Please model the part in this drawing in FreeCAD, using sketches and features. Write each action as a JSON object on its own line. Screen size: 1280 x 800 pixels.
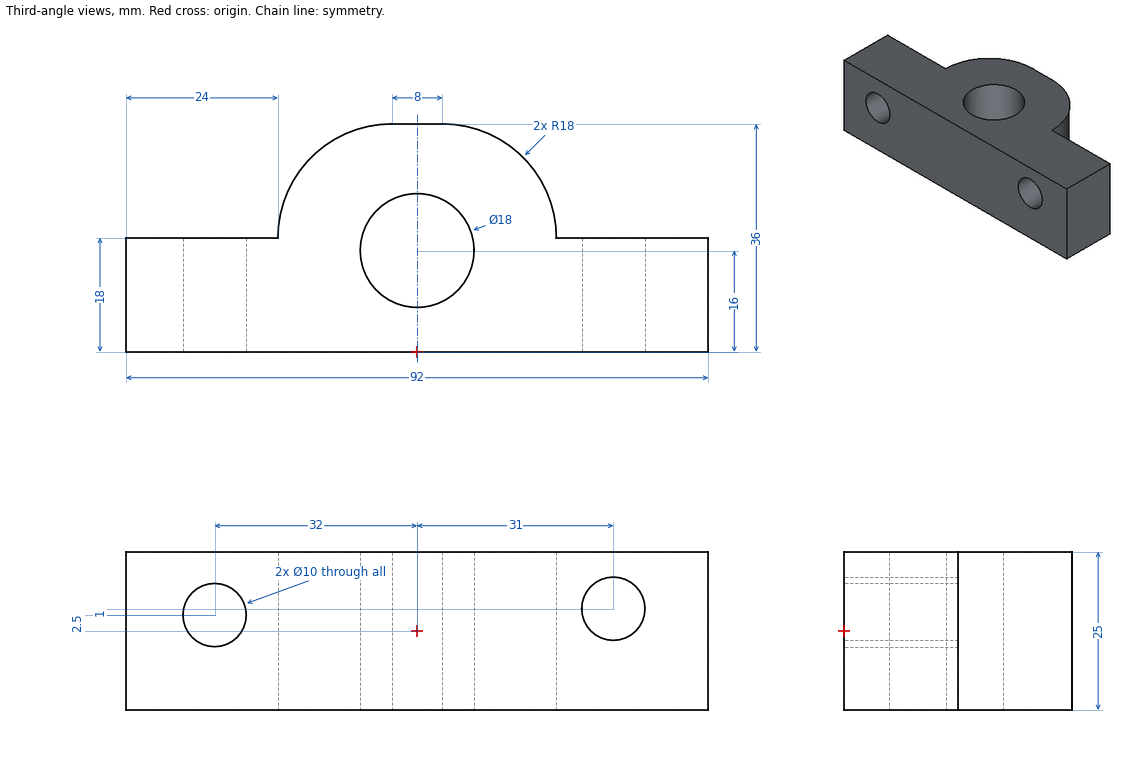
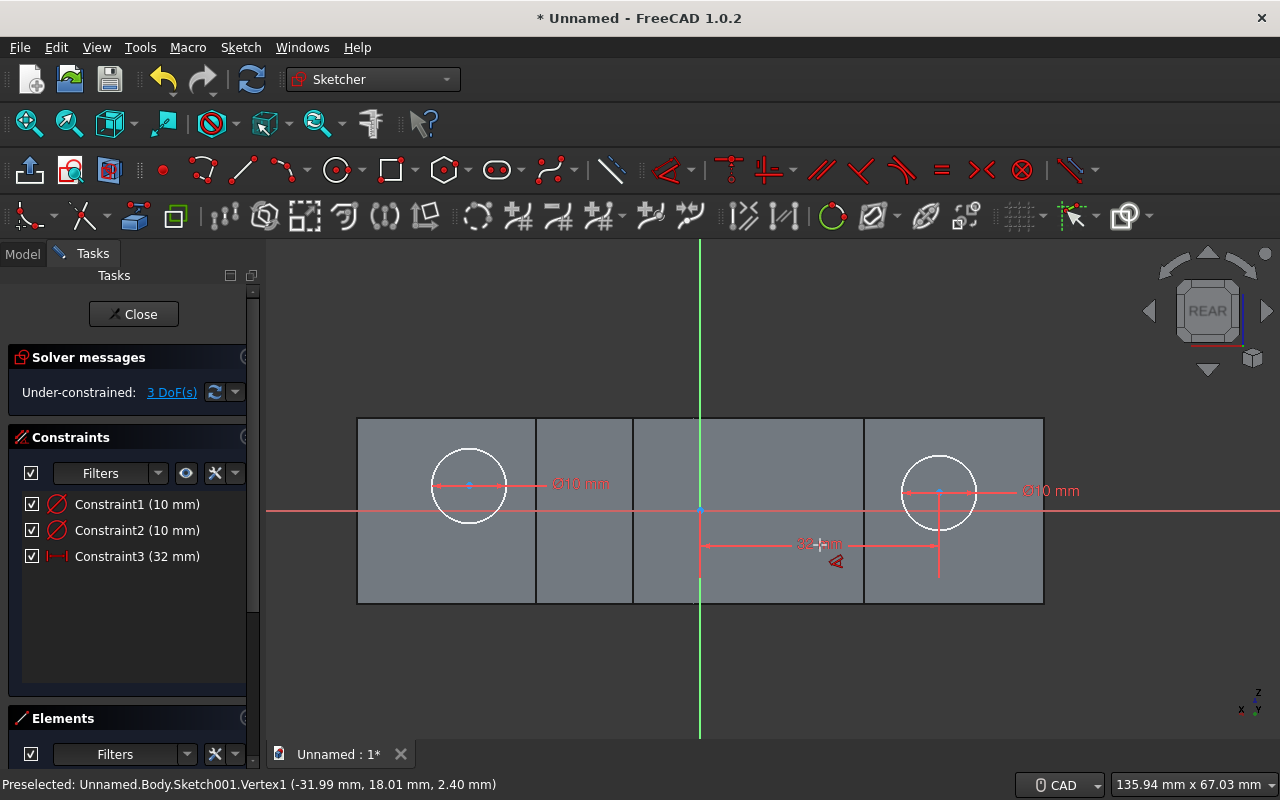
{"action": "left_click", "coordinate": [469, 486]}
{"action": "left_click", "coordinate": [585, 545]}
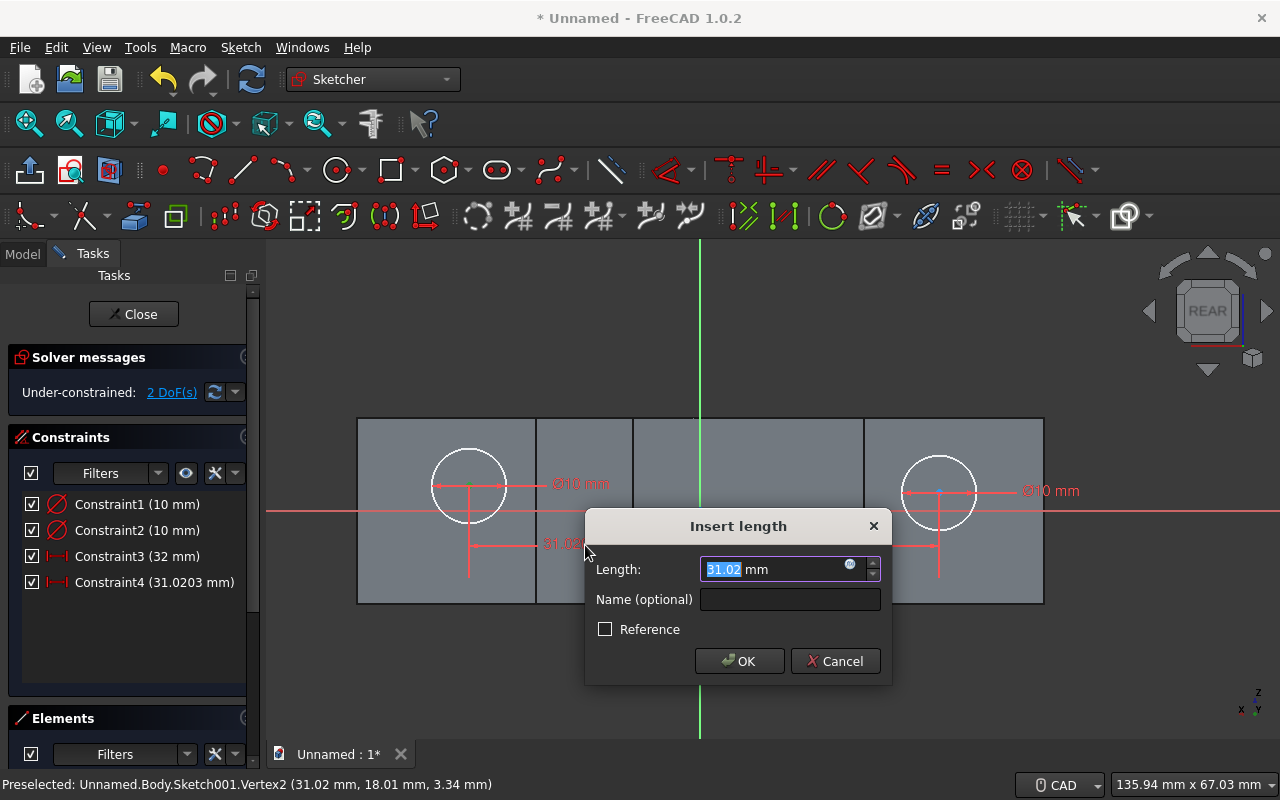
{"action": "type", "text": "31"}
{"action": "key", "text": "Return"}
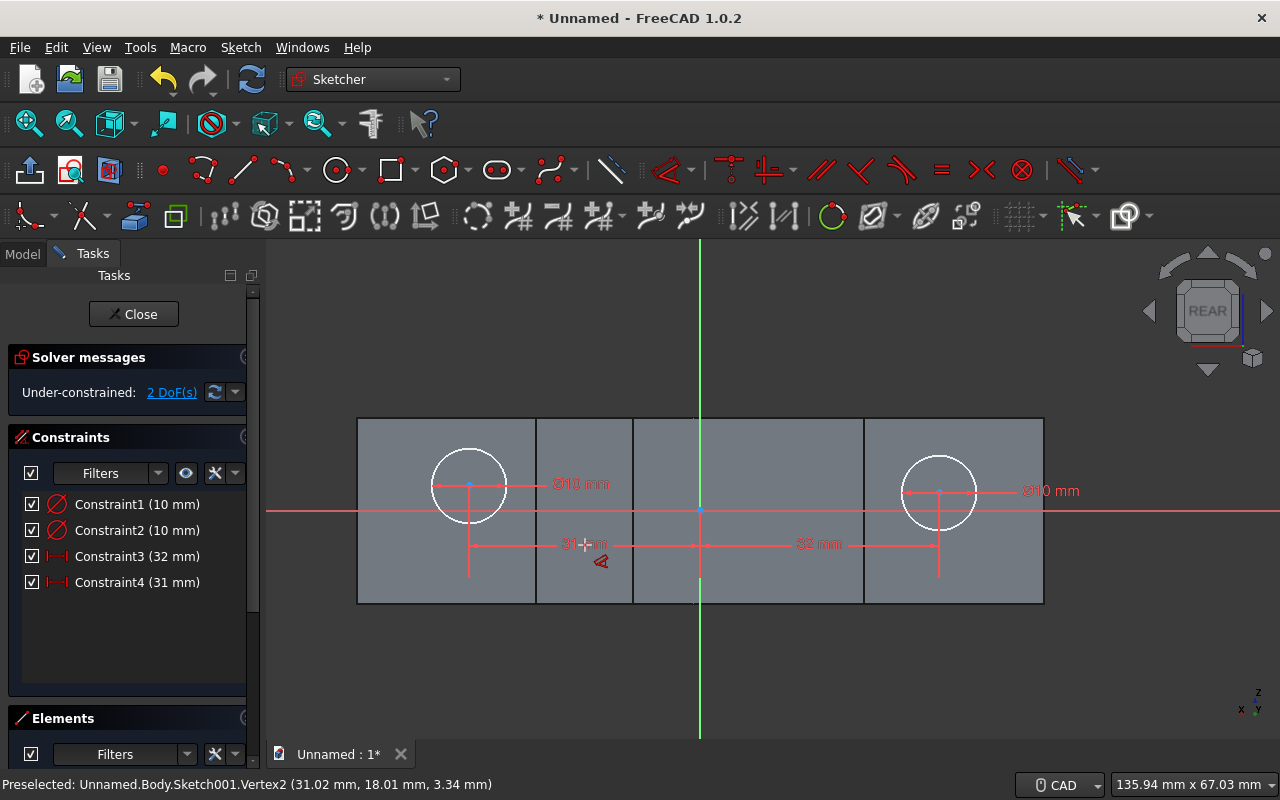
{"action": "scroll", "coordinate": [939, 493], "scroll_direction": "up", "scroll_amount": 9}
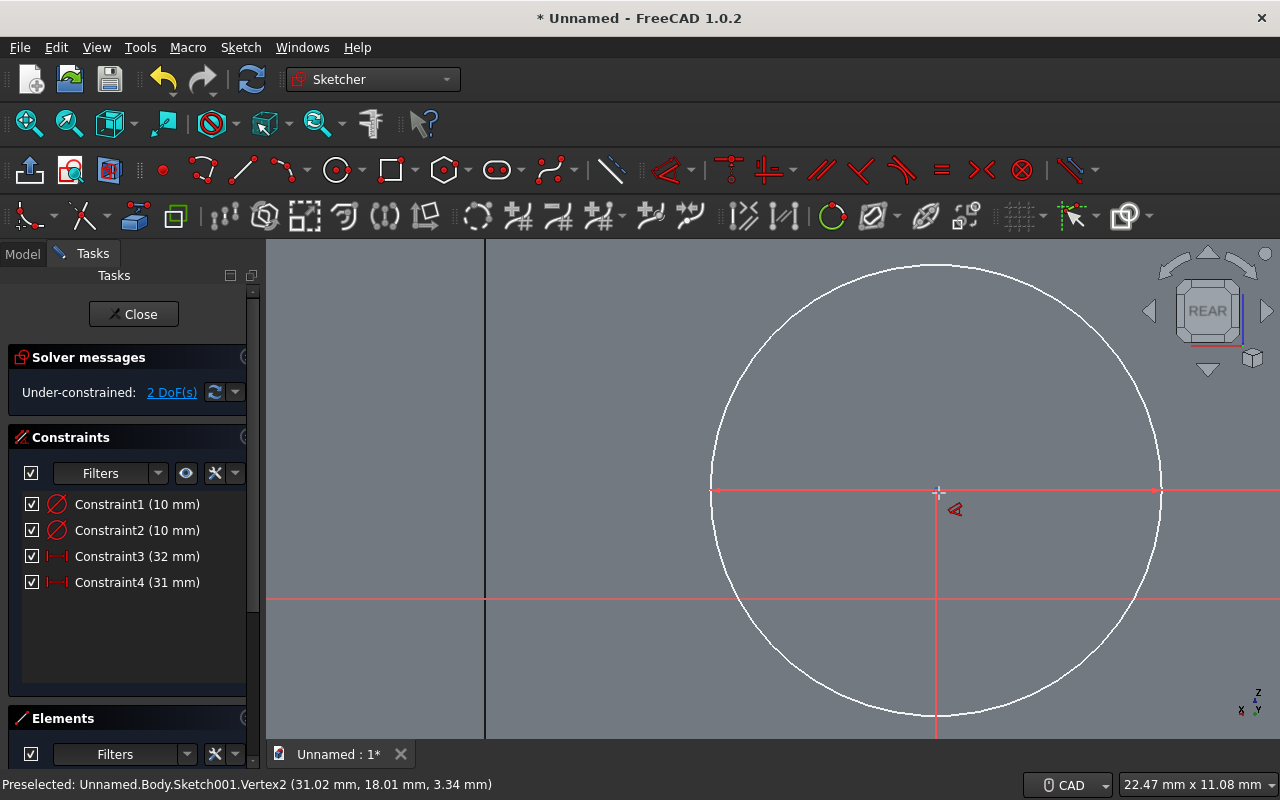
{"action": "left_click", "coordinate": [936, 490]}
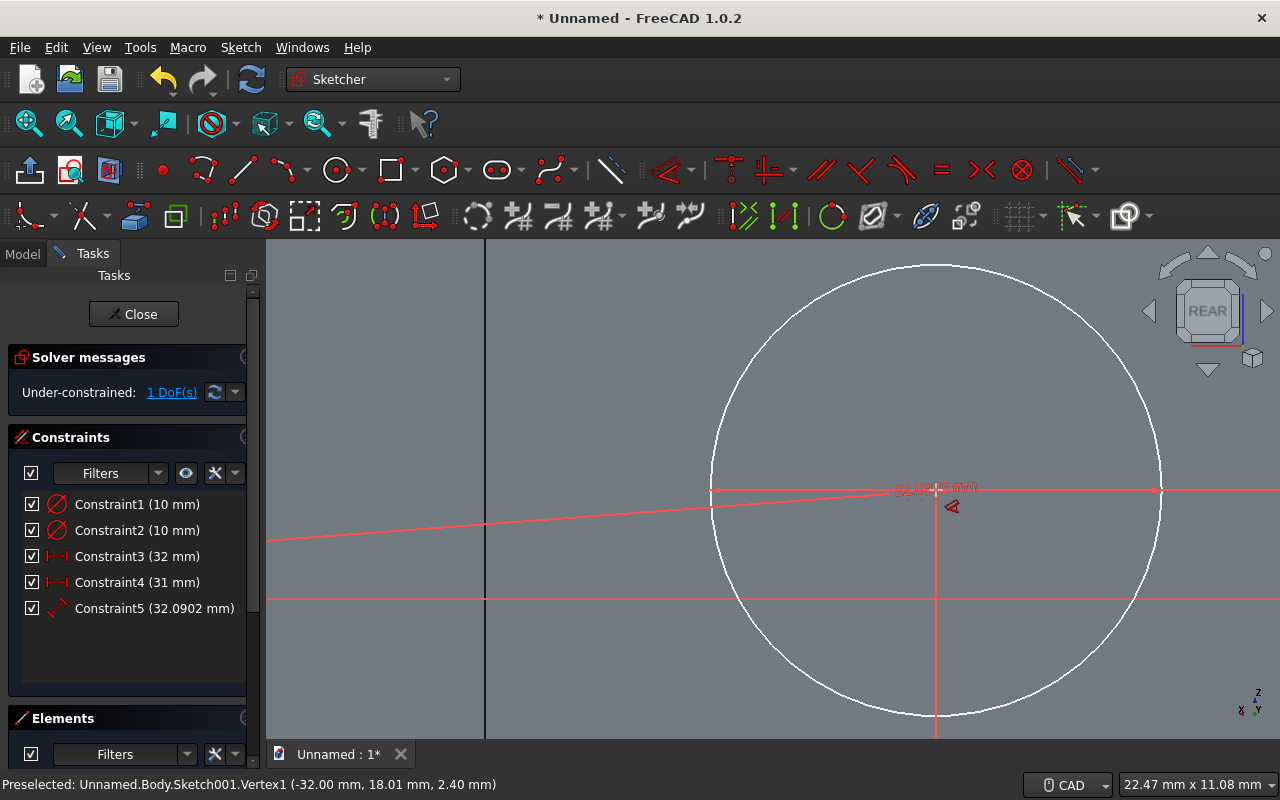
{"action": "scroll", "coordinate": [940, 494], "scroll_direction": "down", "scroll_amount": 9}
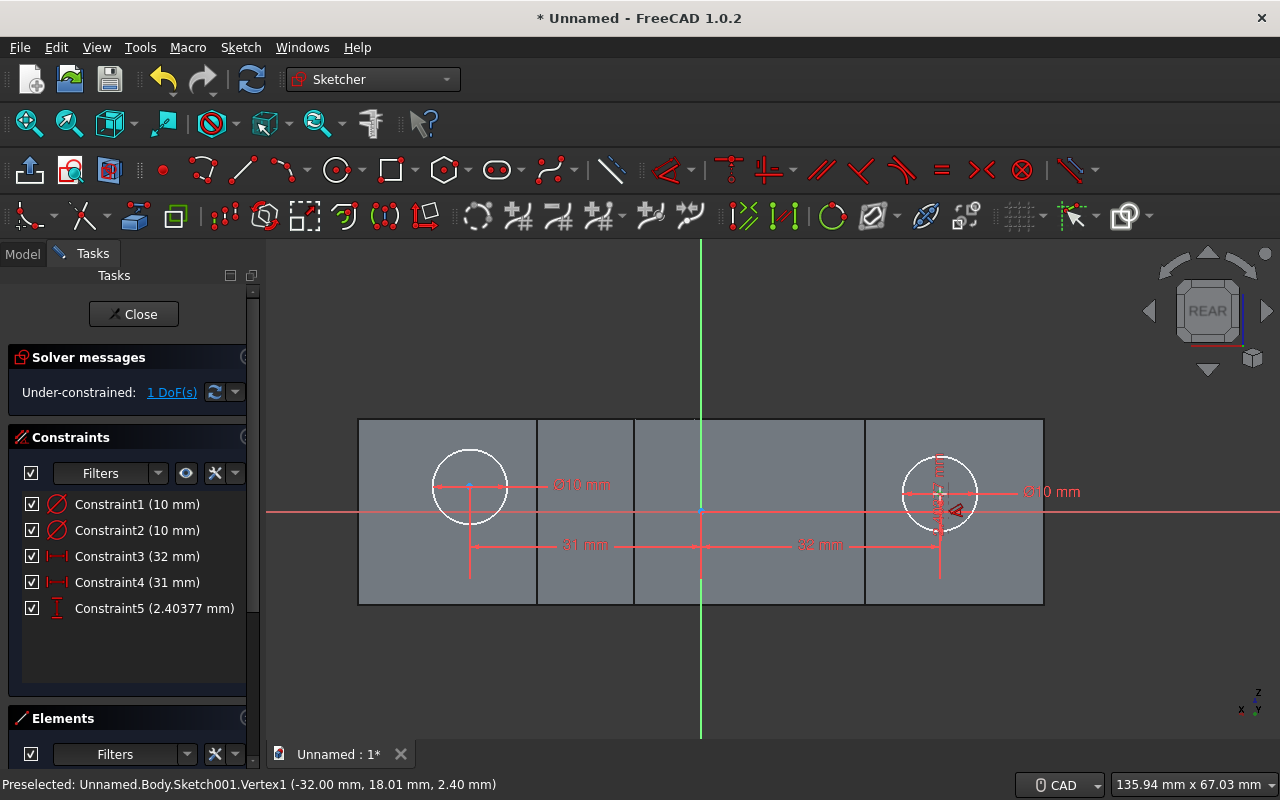
{"action": "scroll", "coordinate": [470, 487], "scroll_direction": "up", "scroll_amount": 9}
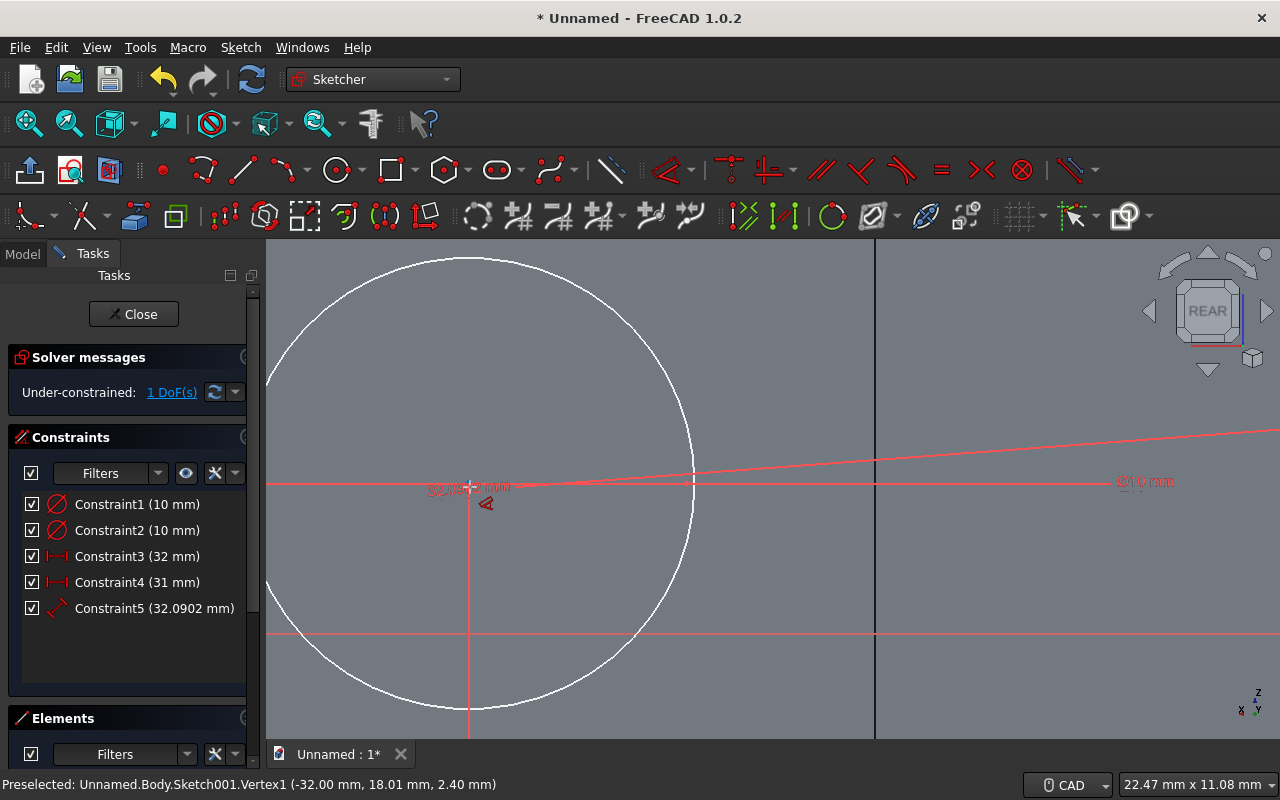
{"action": "left_click", "coordinate": [469, 484]}
{"action": "left_click", "coordinate": [435, 505]}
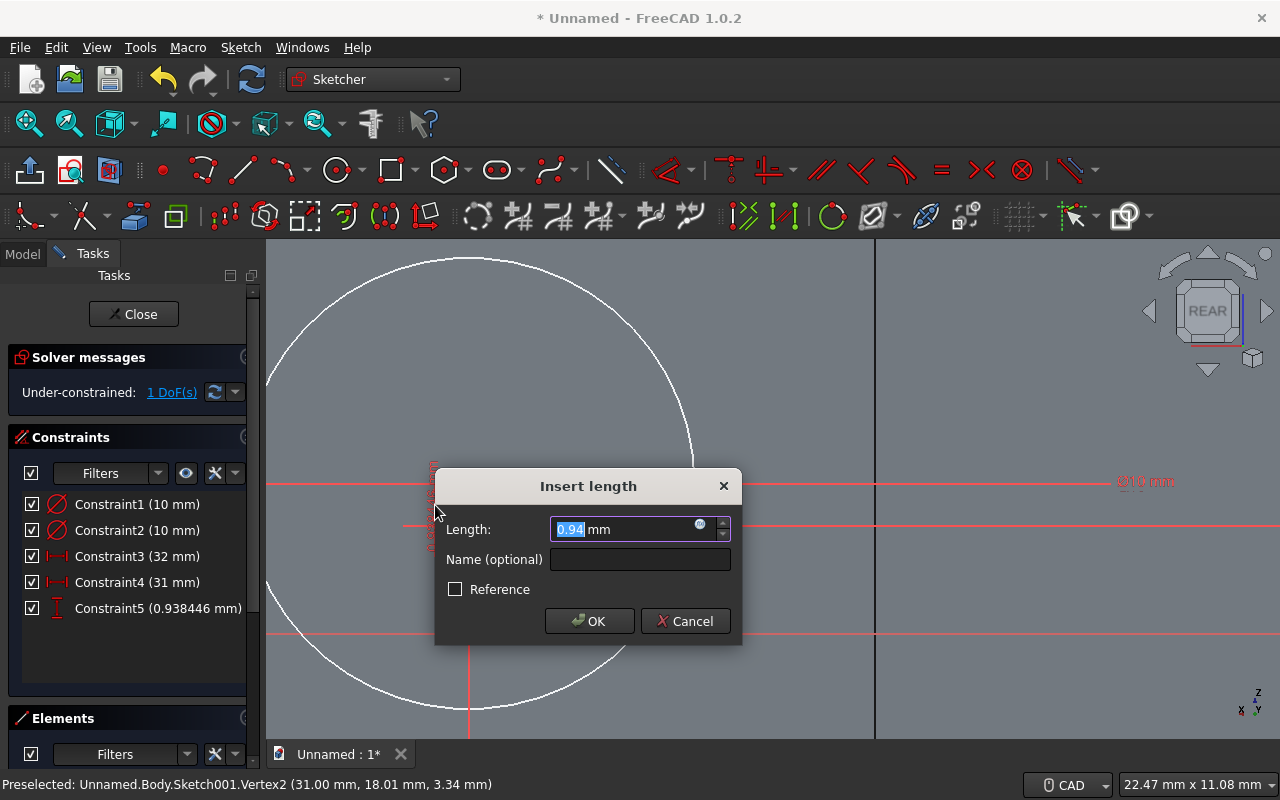
{"action": "type", "text": "1"}
{"action": "key", "text": "Return"}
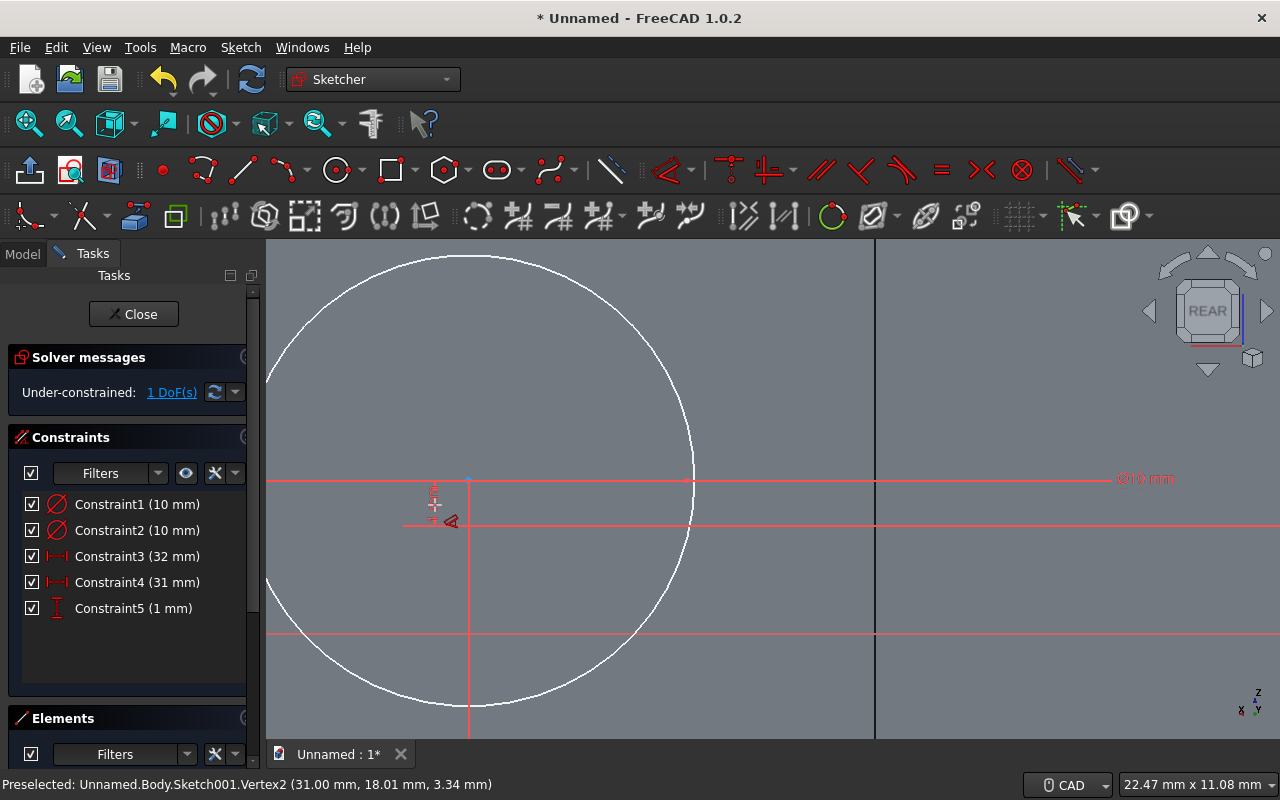
{"action": "scroll", "coordinate": [470, 487], "scroll_direction": "down", "scroll_amount": 9}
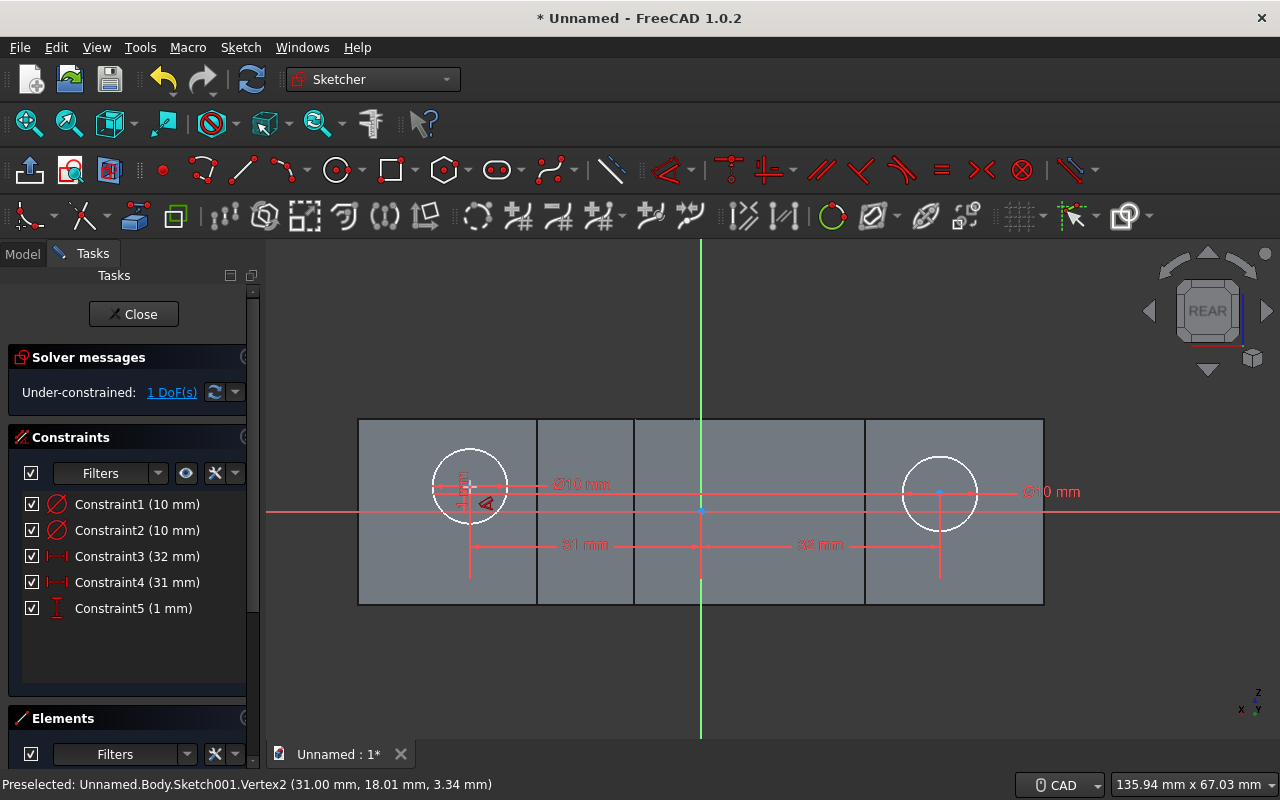
{"action": "scroll", "coordinate": [940, 494], "scroll_direction": "up", "scroll_amount": 4}